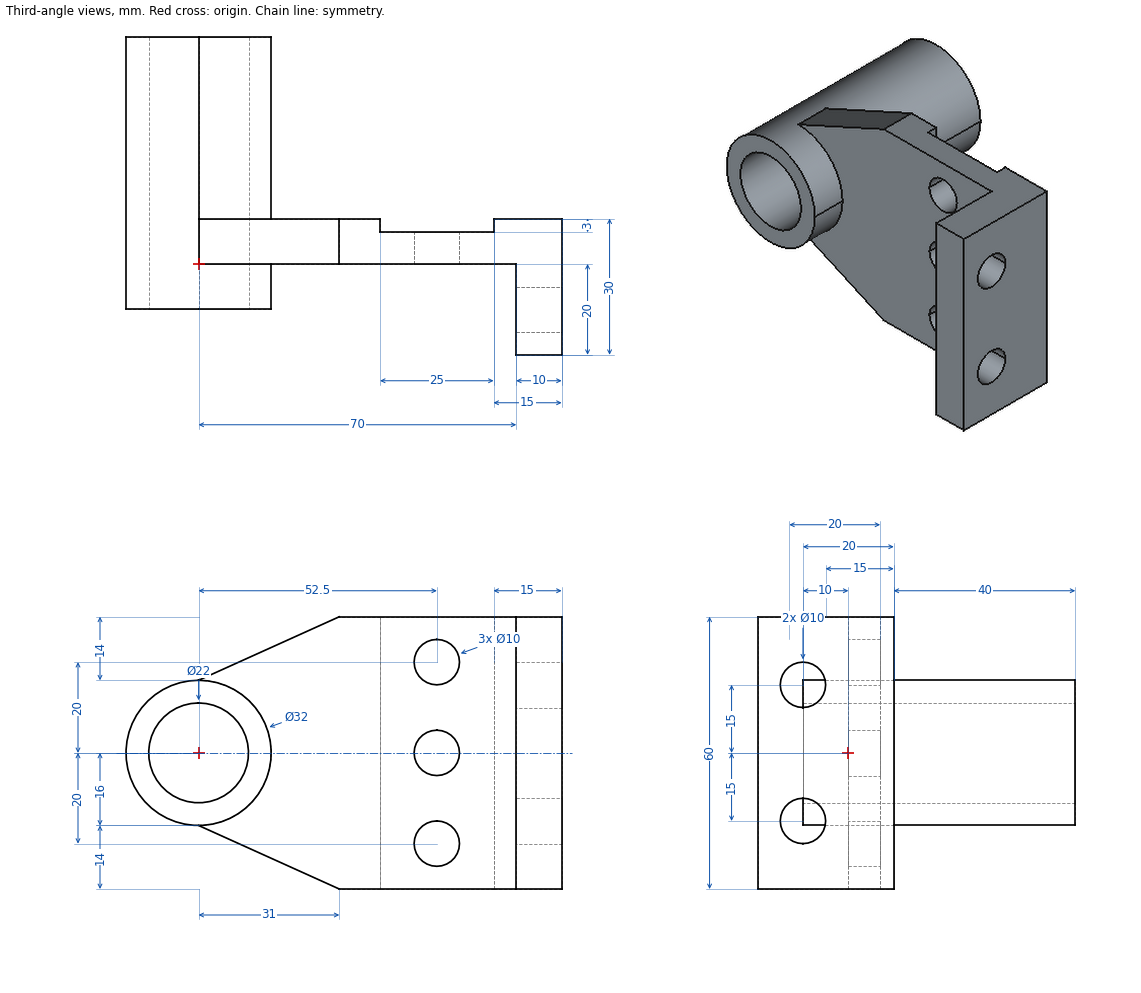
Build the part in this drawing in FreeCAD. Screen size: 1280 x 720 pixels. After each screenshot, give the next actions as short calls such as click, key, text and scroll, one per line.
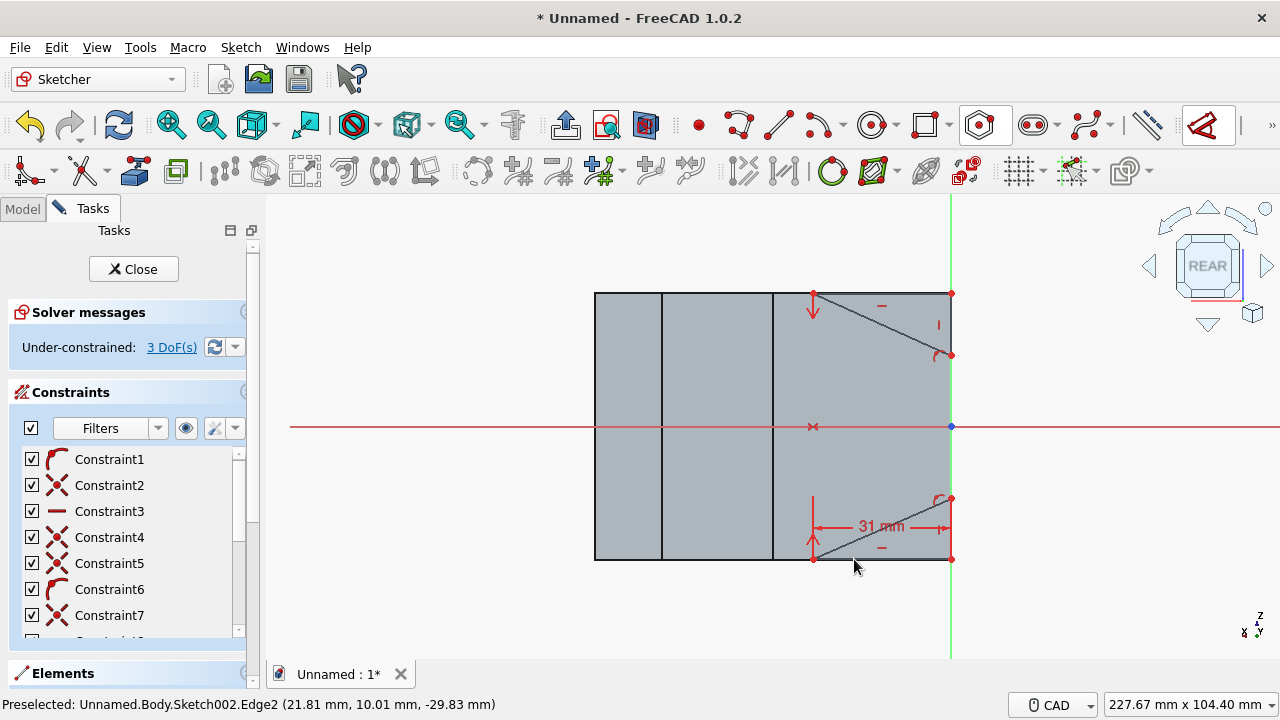
click(951, 541)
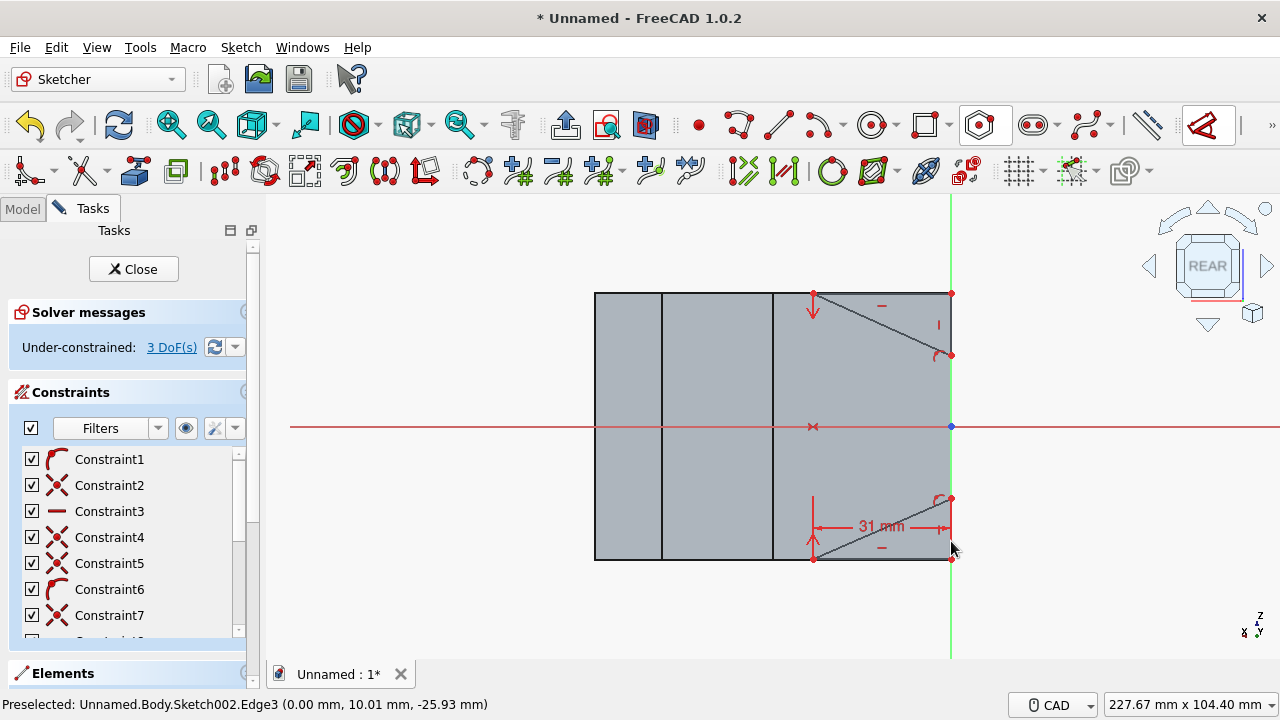
click(1230, 126)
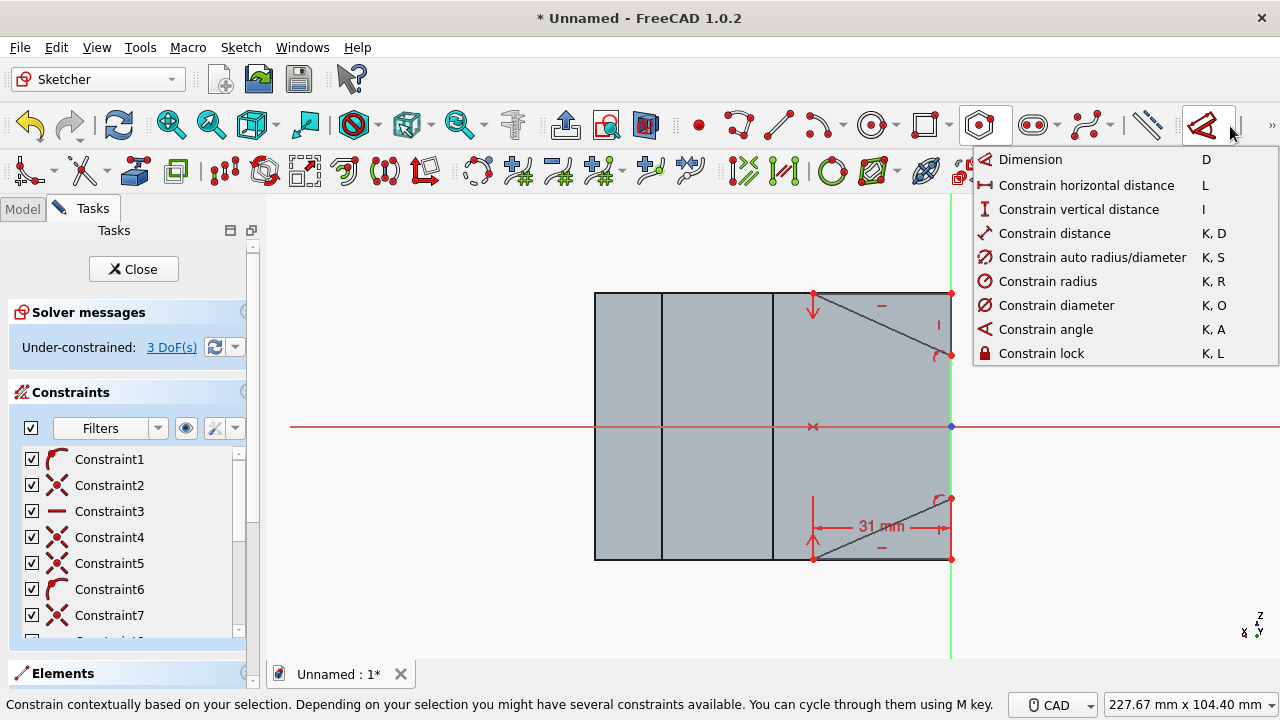
click(1126, 209)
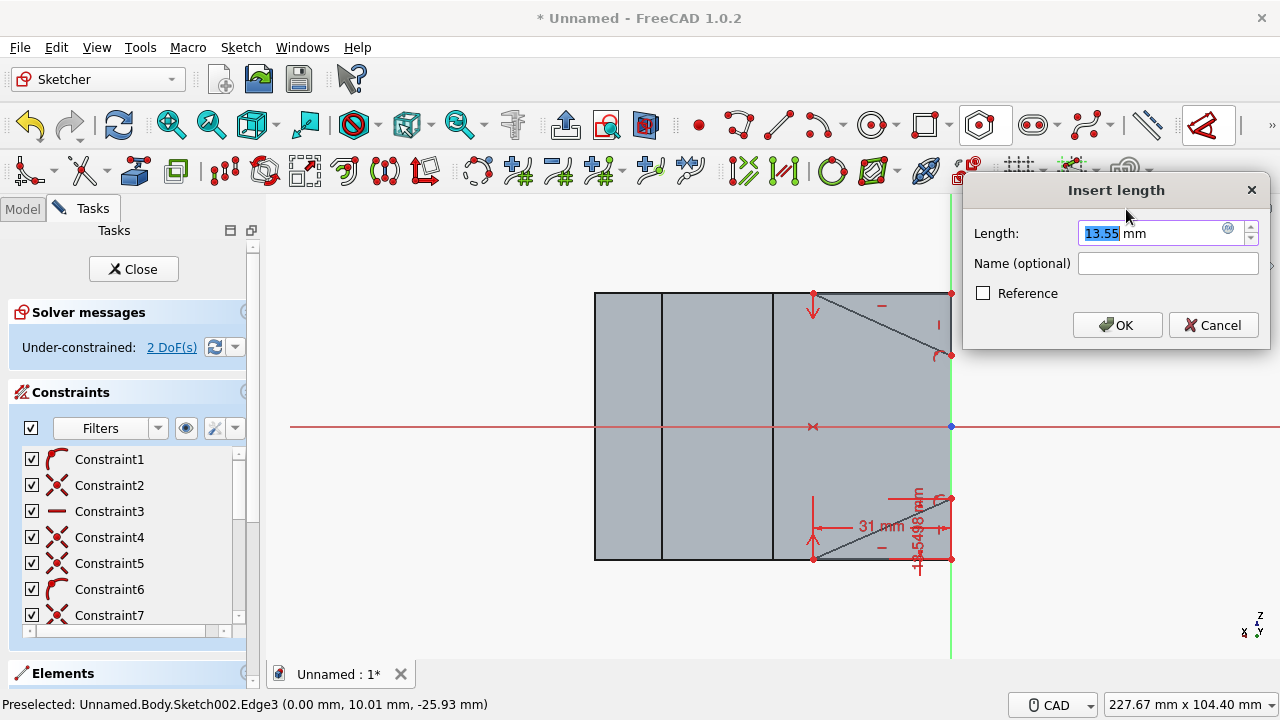
text(14)
key(Return)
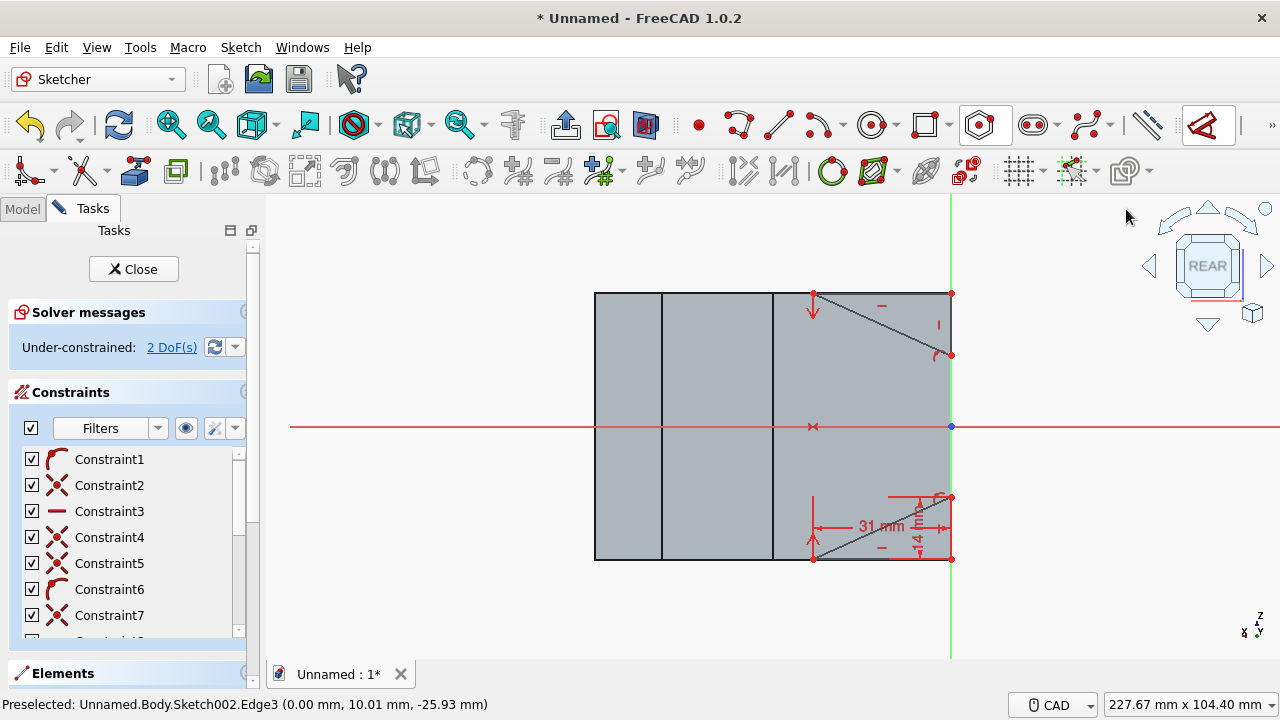
click(951, 337)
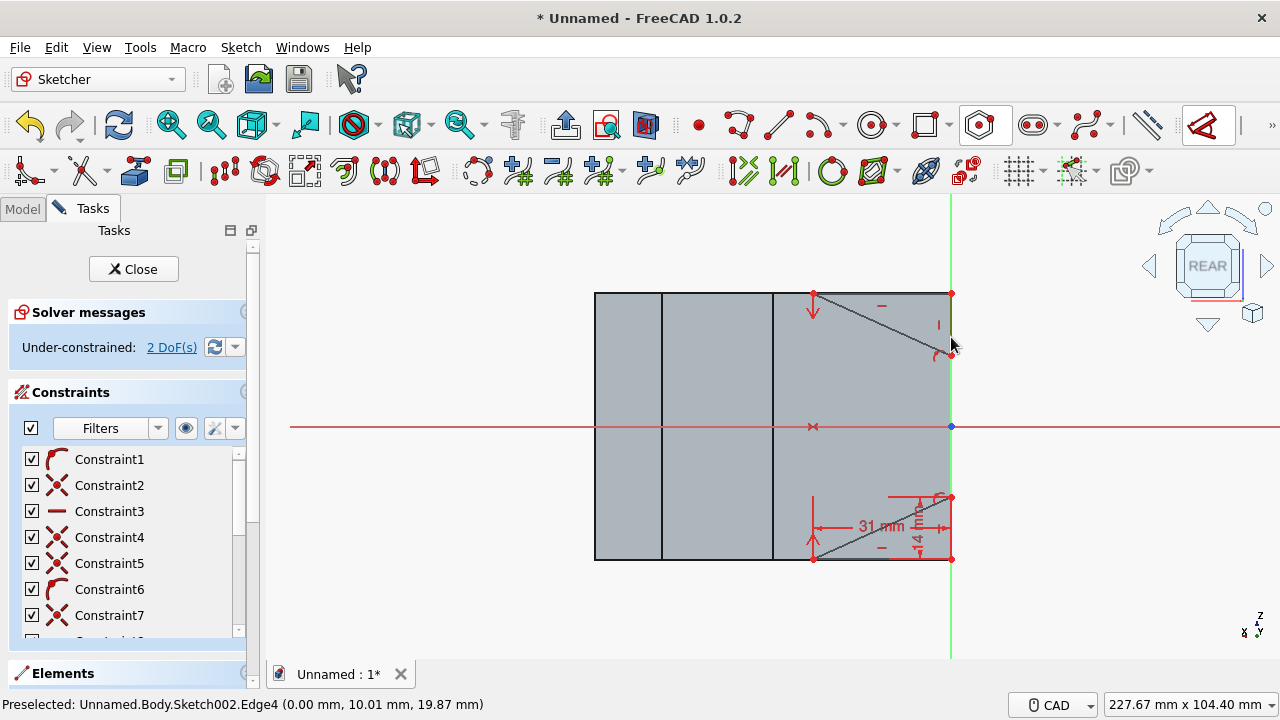
click(1230, 126)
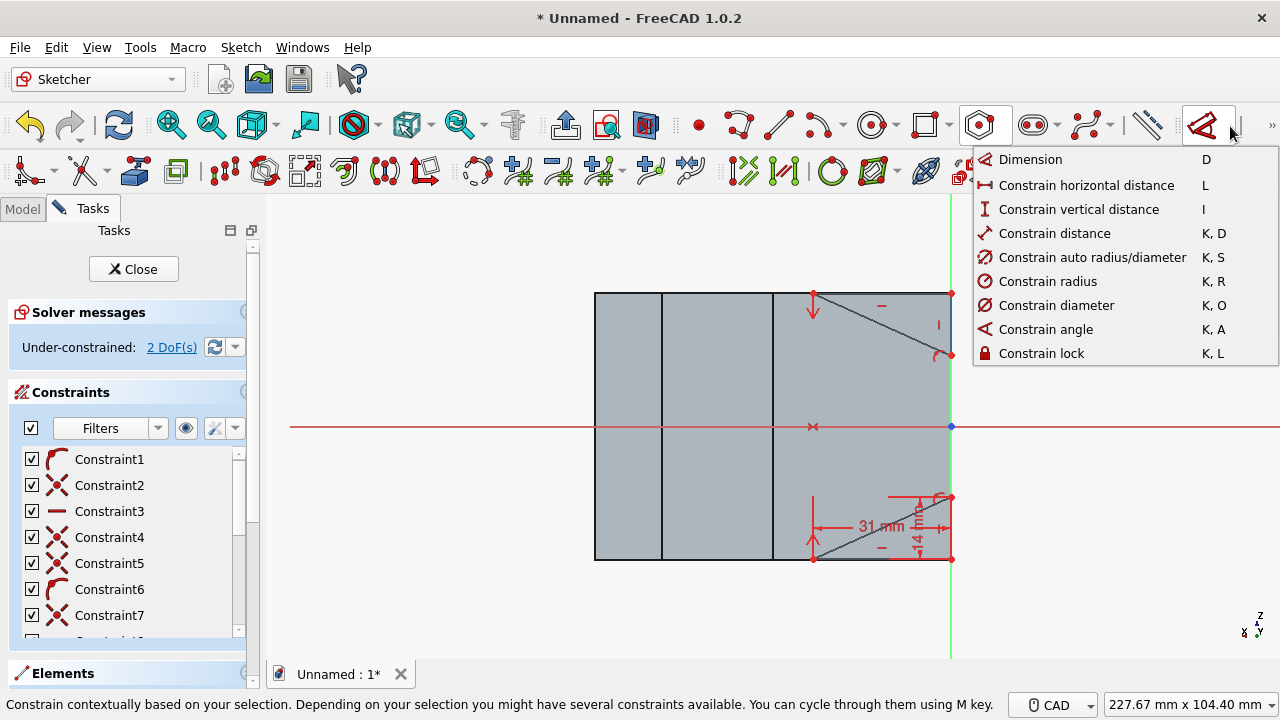
click(1126, 209)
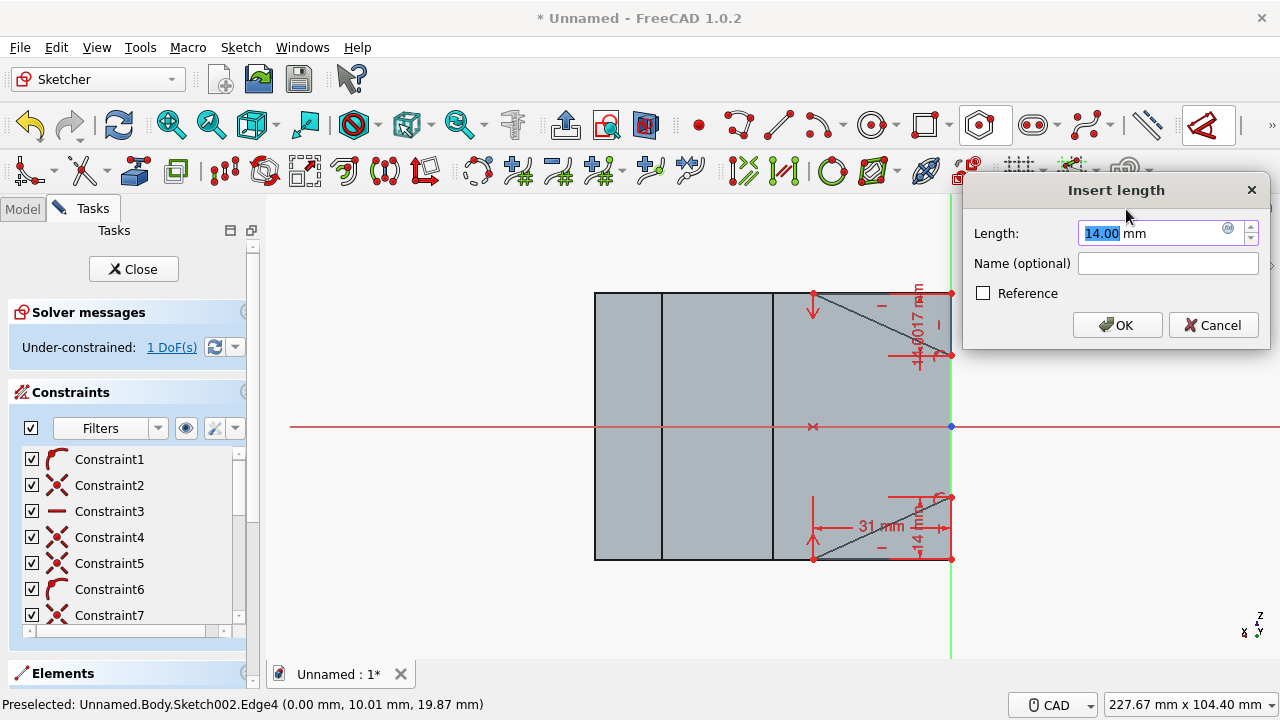
text(14)
key(Return)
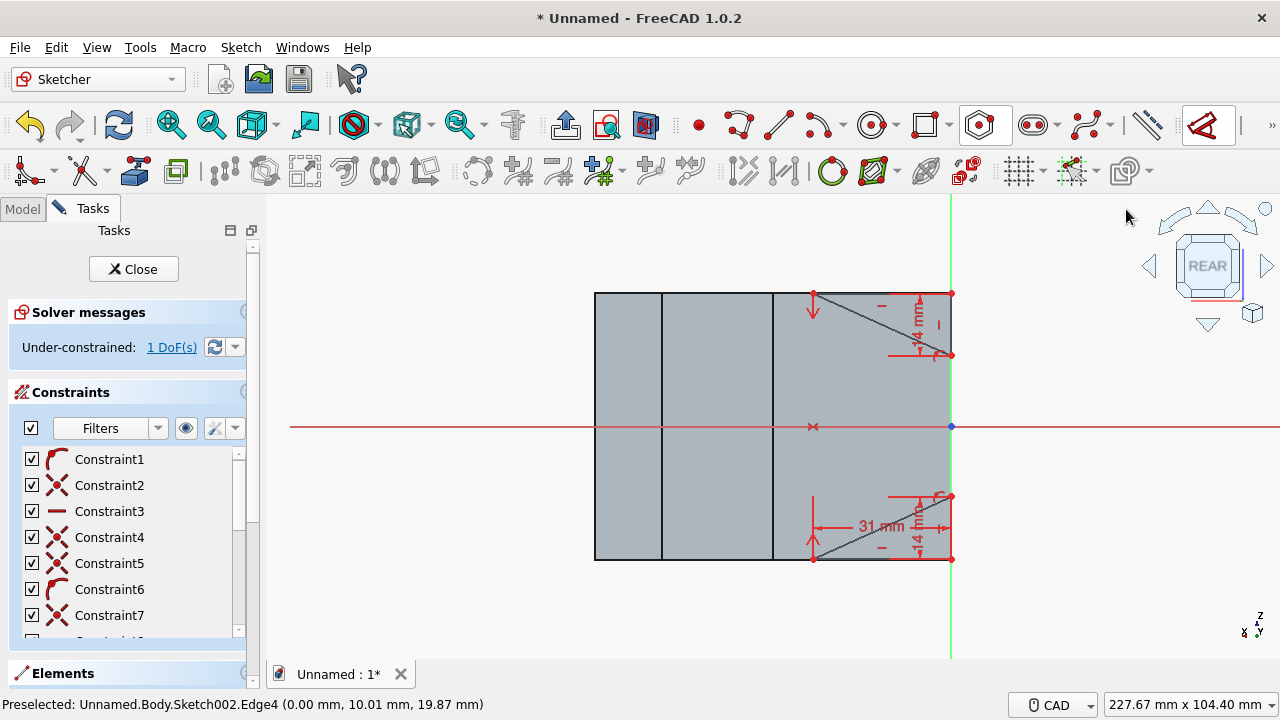
click(951, 497)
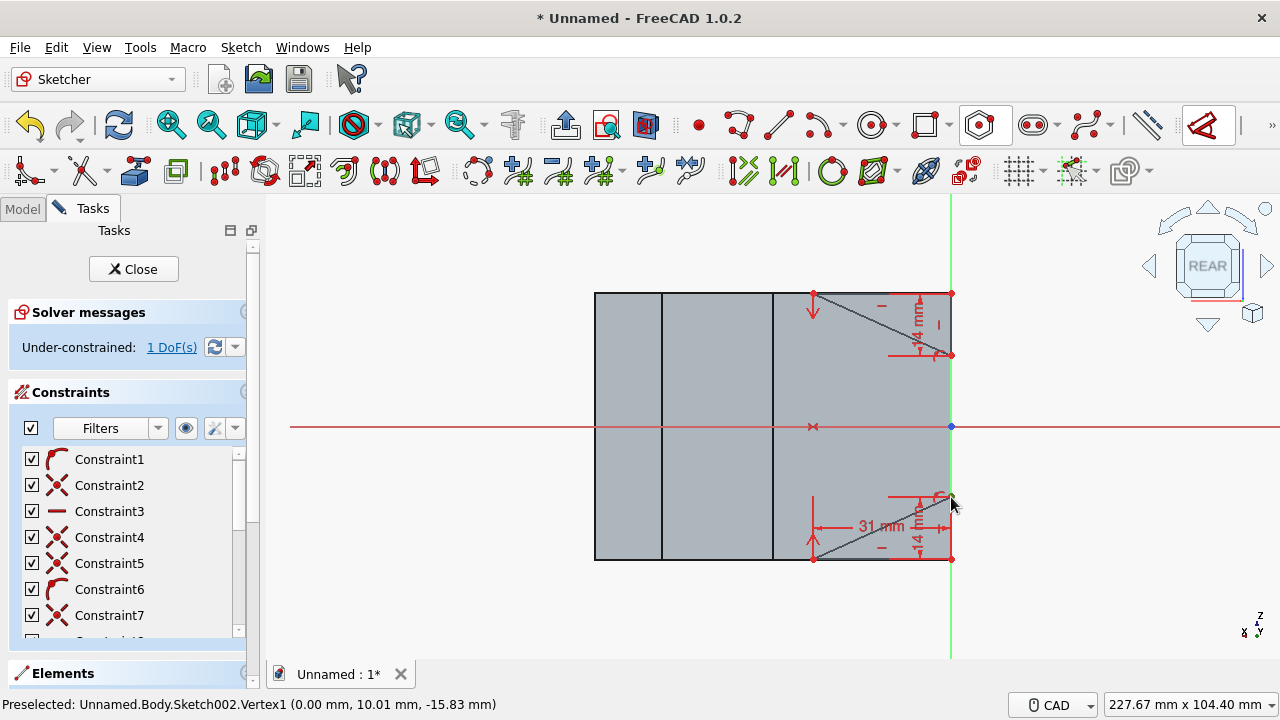
click(1230, 126)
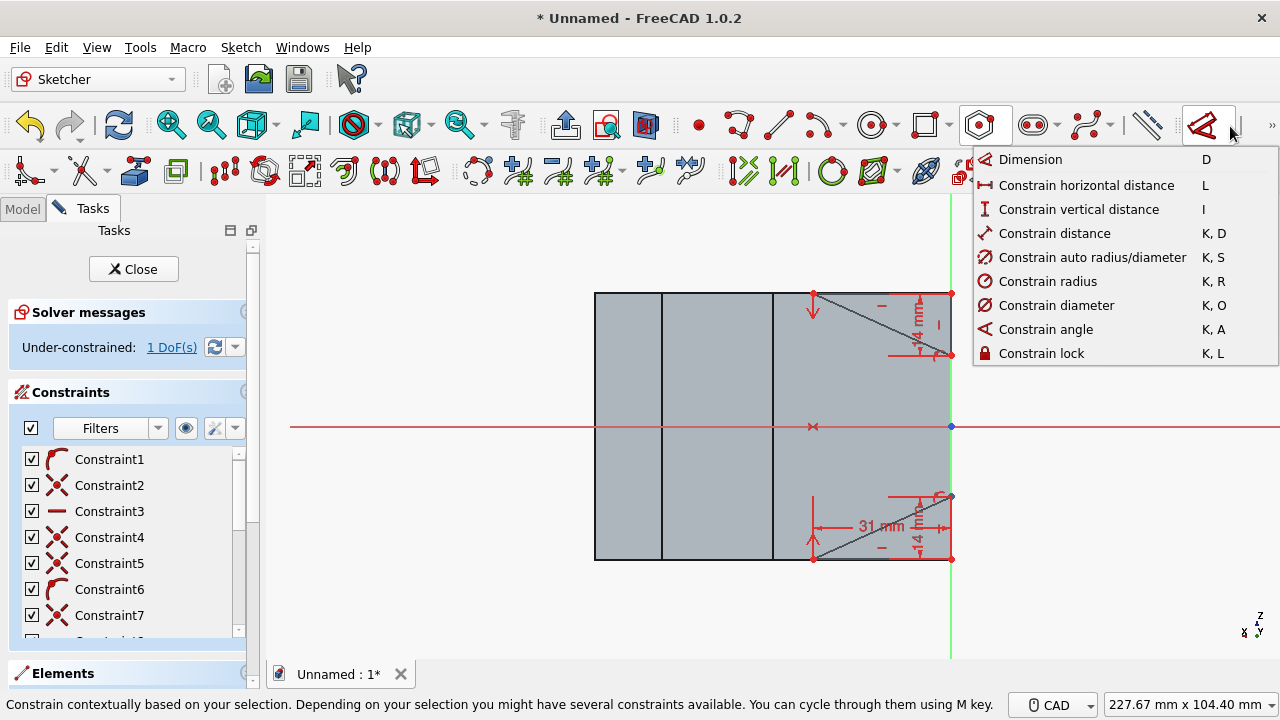
click(1126, 209)